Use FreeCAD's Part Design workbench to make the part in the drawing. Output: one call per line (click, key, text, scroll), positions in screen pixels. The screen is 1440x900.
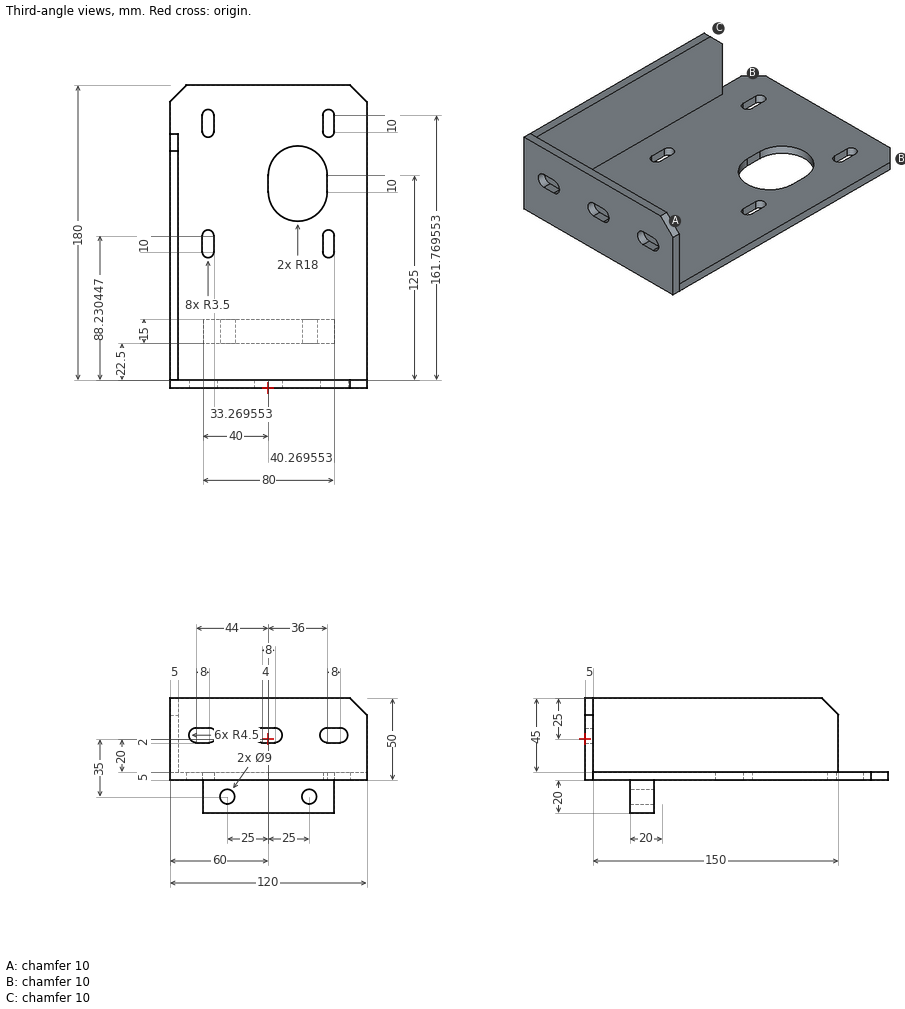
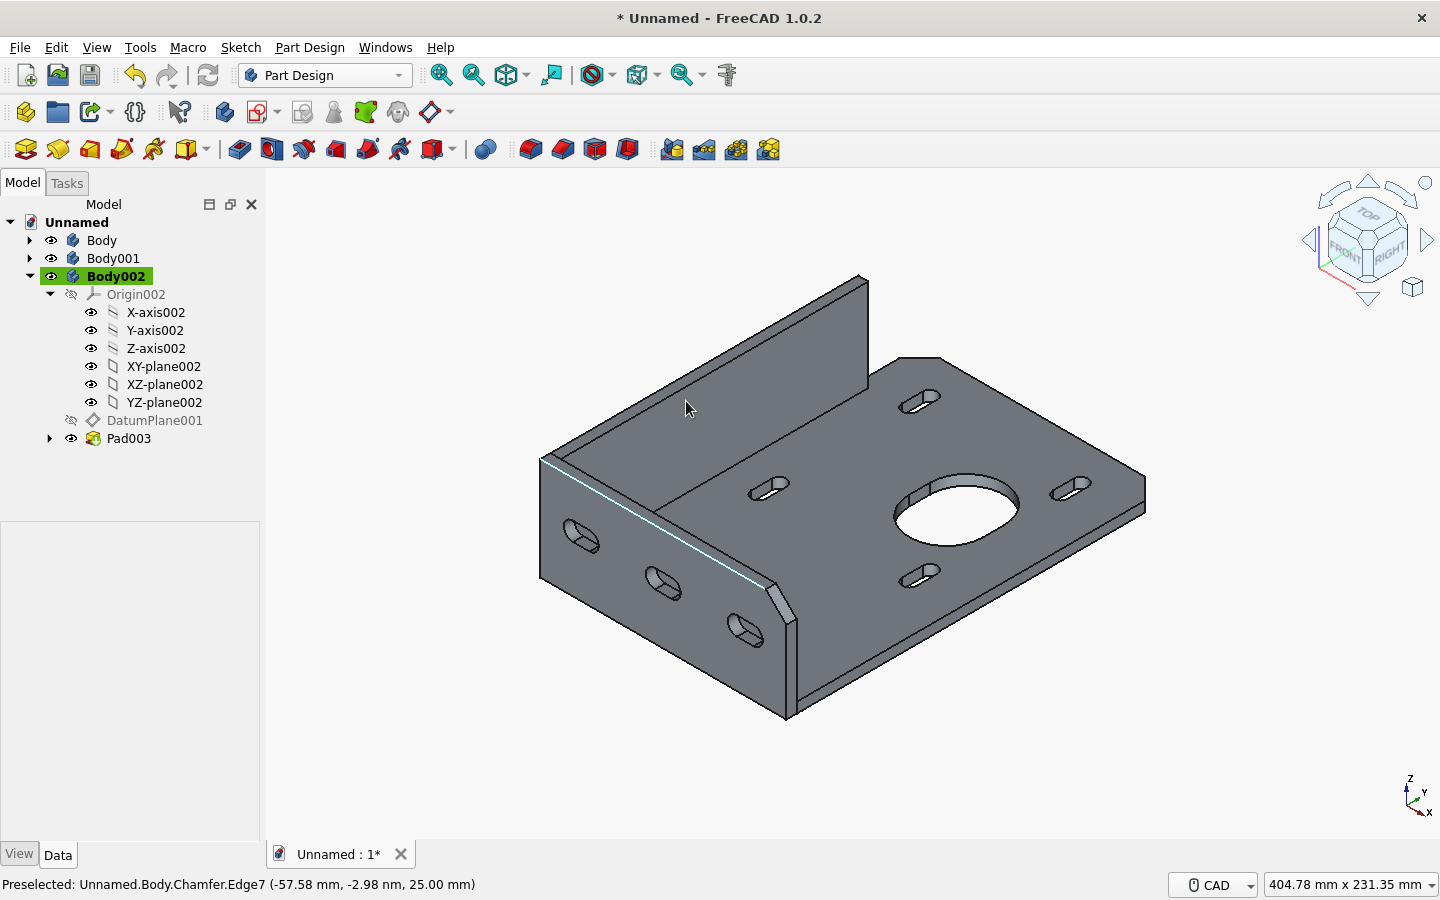
scroll(863, 278, up, 6)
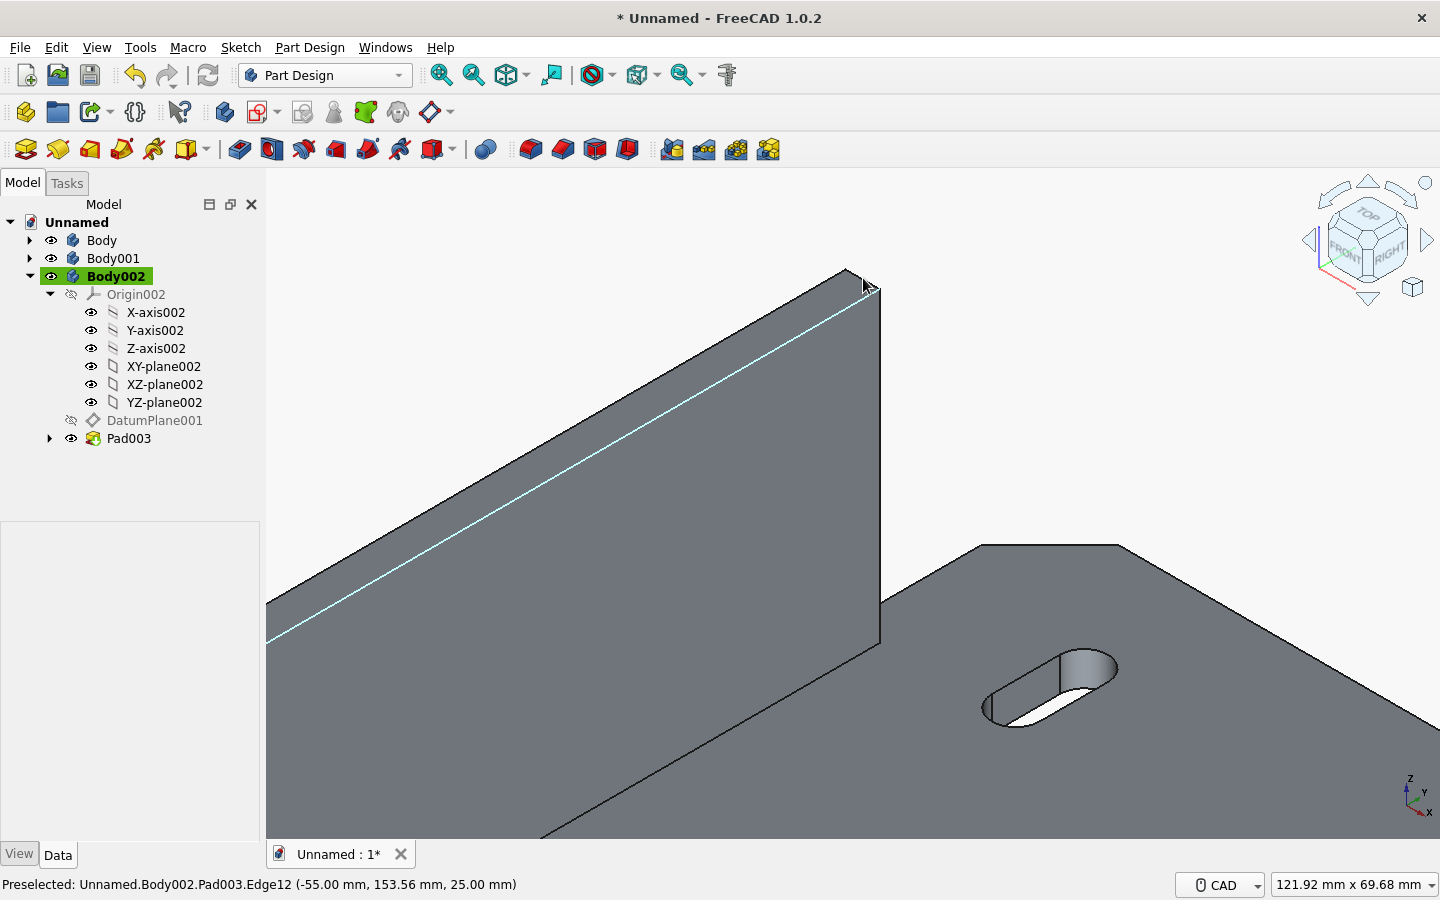
key(v)
key(f)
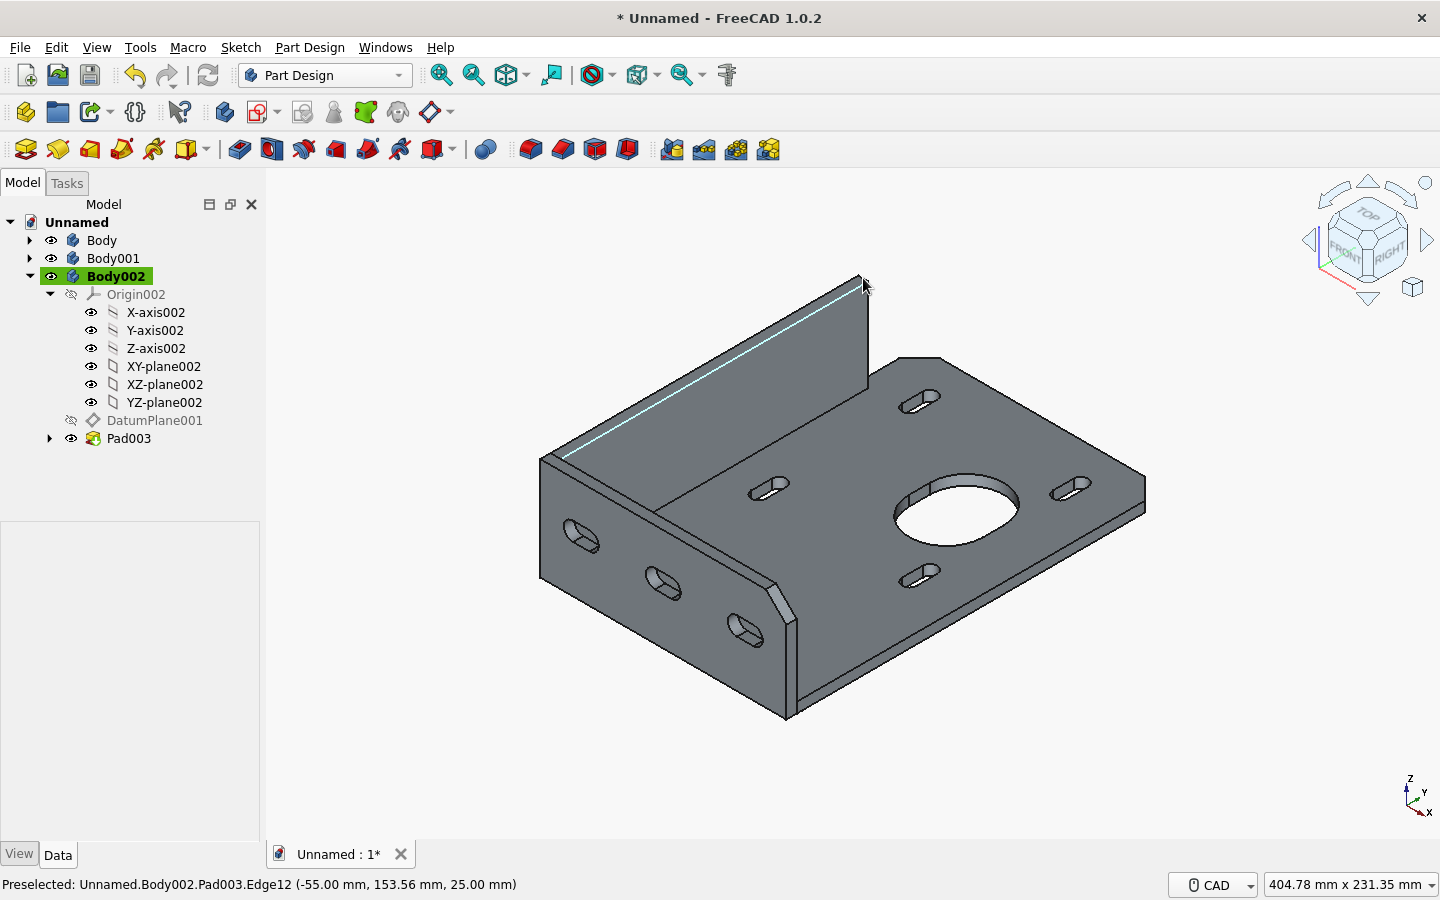
key(2)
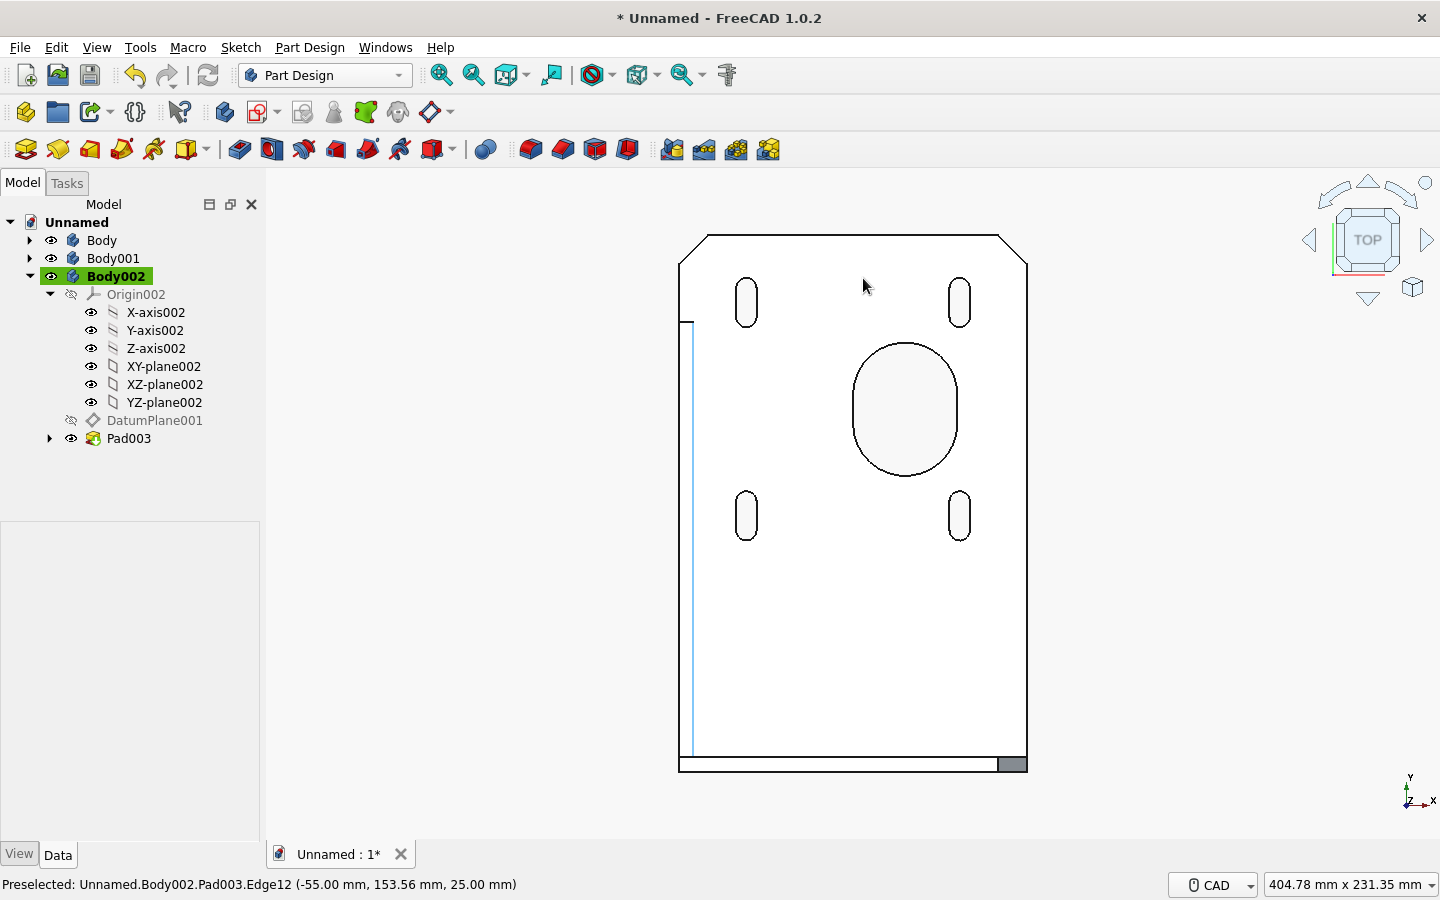
click(686, 321)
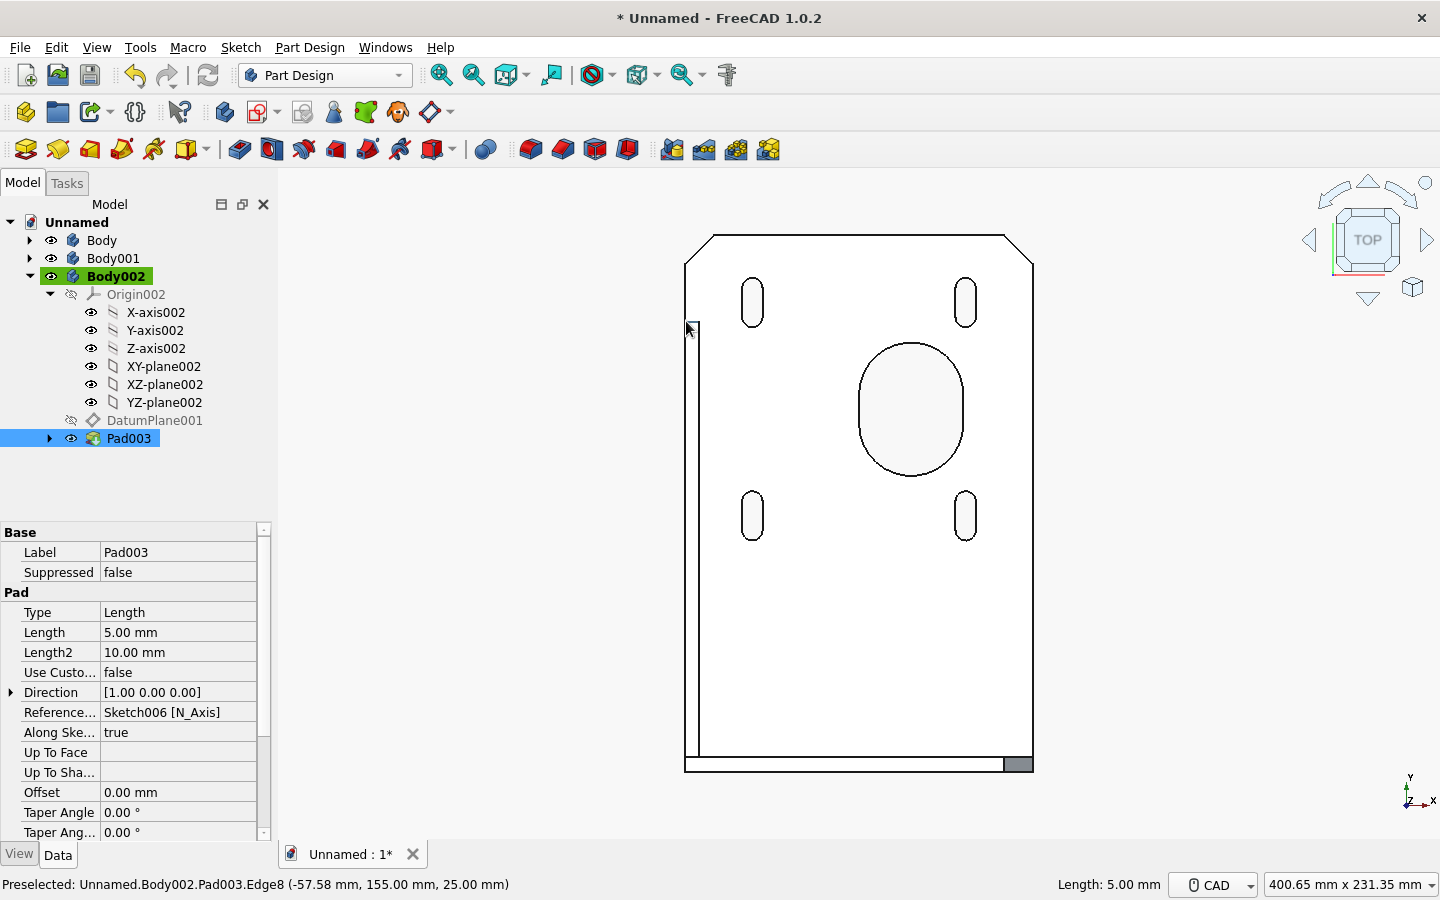
click(564, 150)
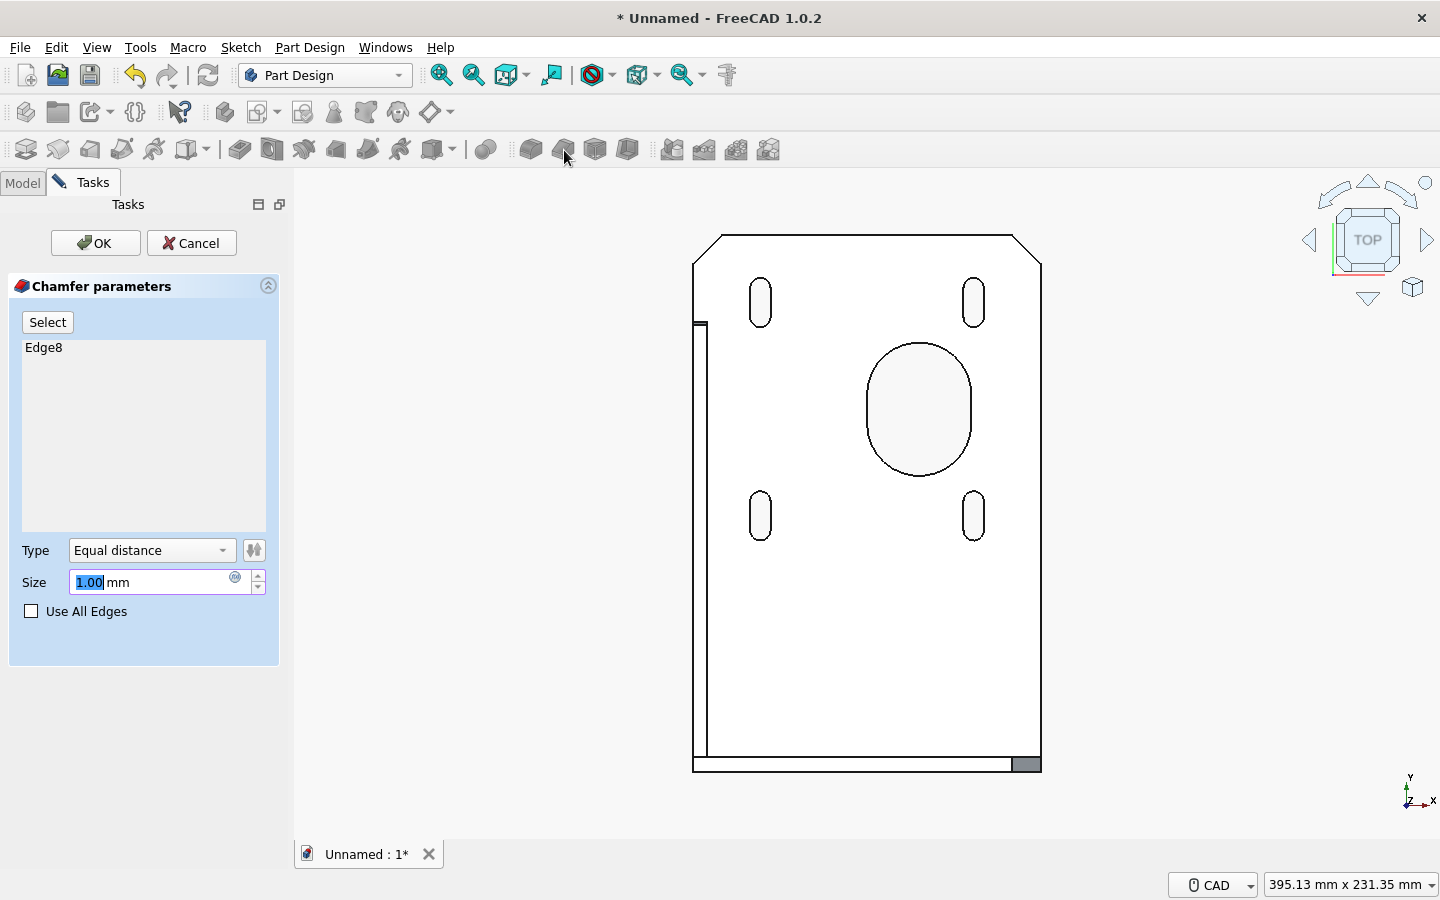
text(10)
key(Tab)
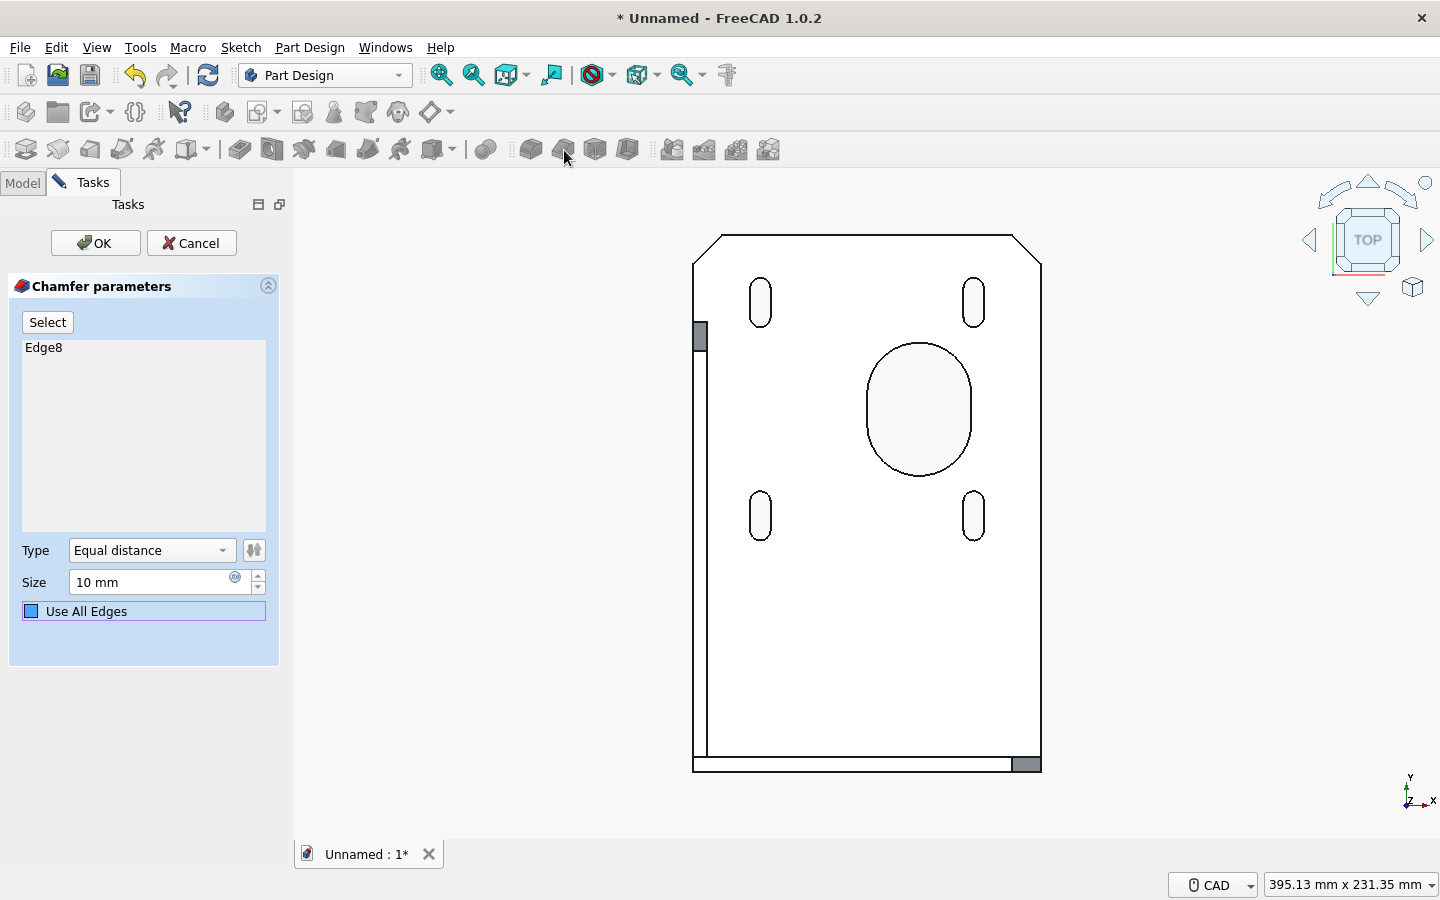
click(96, 243)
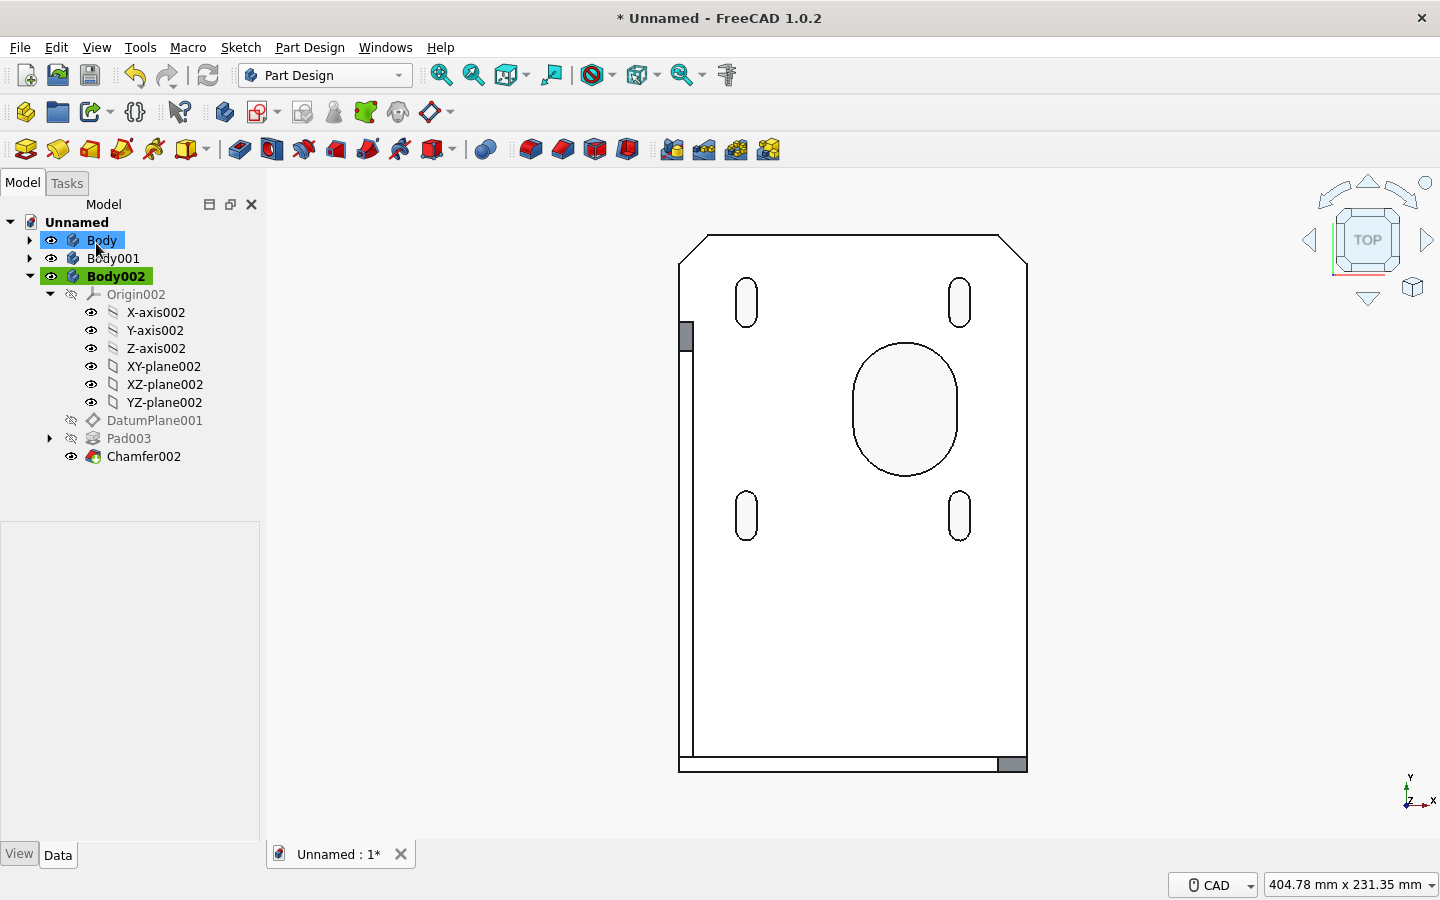
key(0)